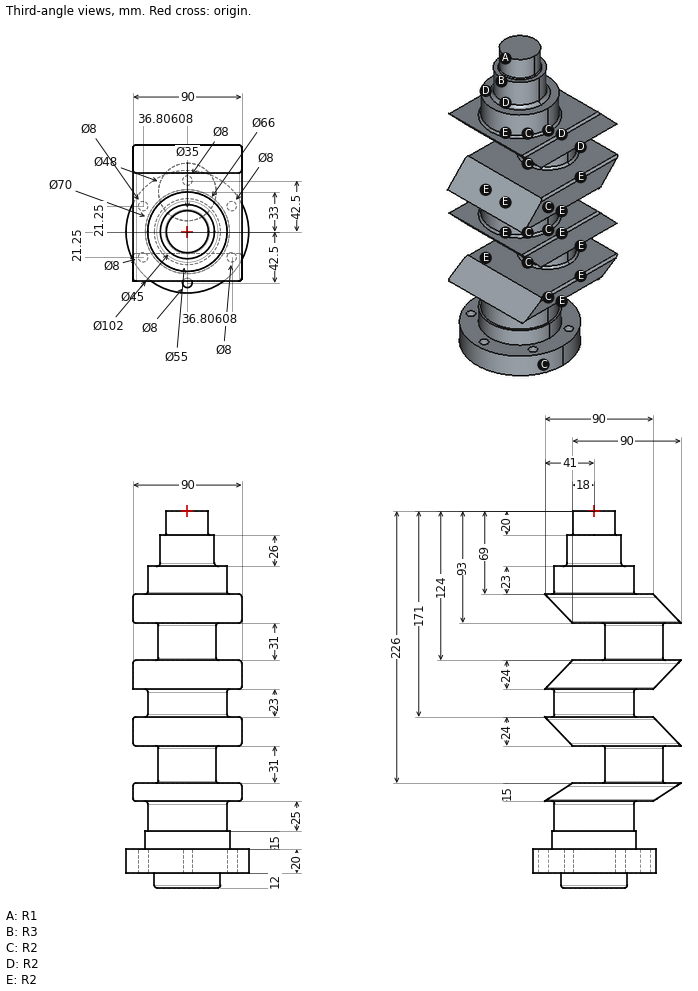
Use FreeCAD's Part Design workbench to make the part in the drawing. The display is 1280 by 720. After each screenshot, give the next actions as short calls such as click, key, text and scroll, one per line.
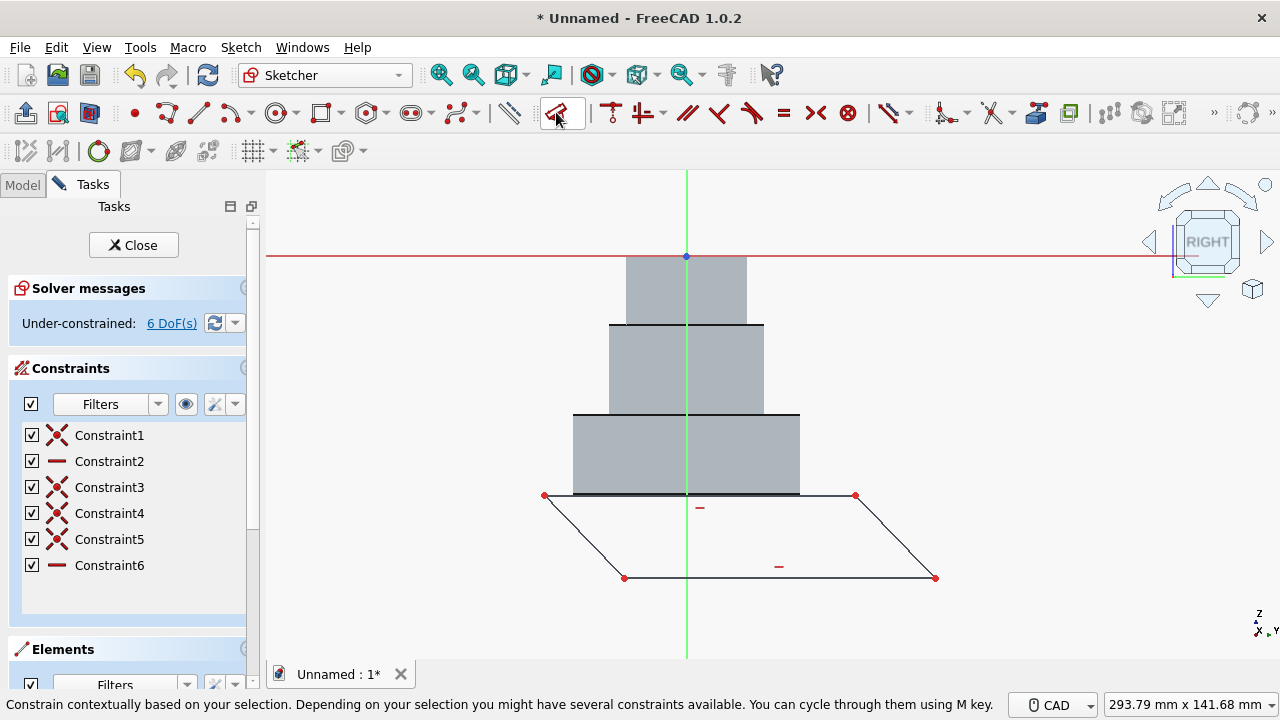
click(718, 578)
click(780, 612)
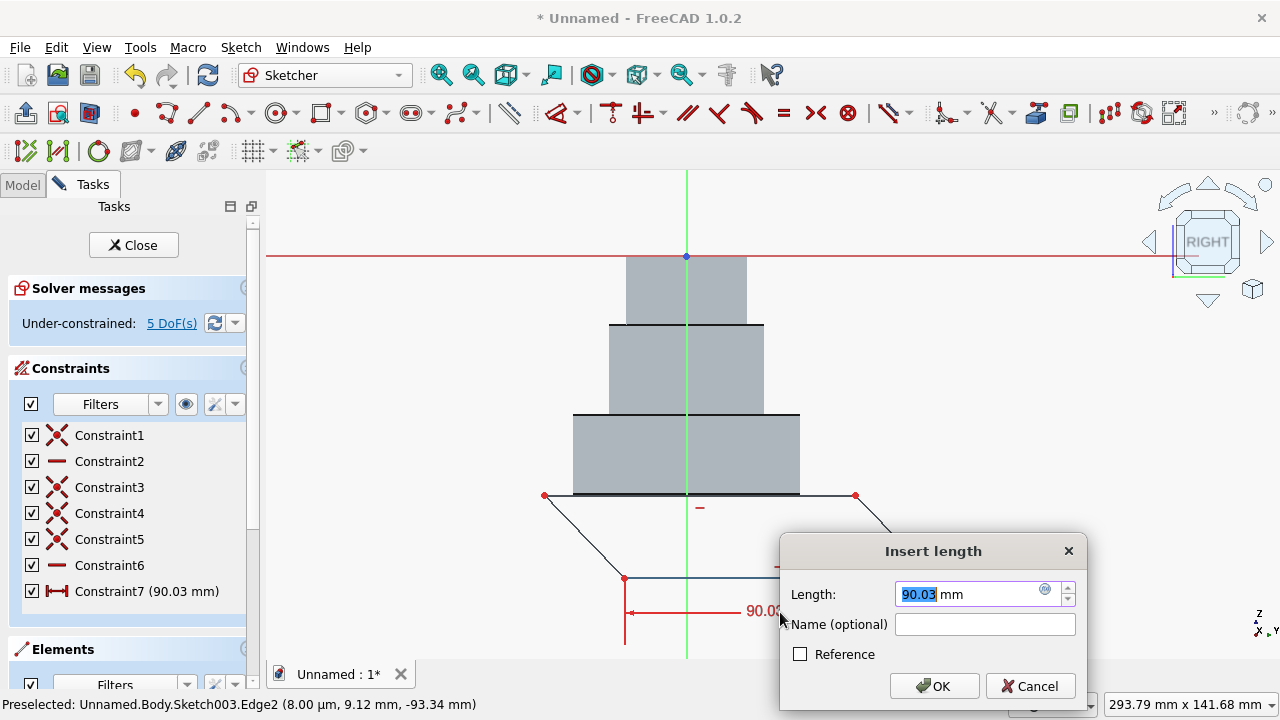
text(90)
key(Return)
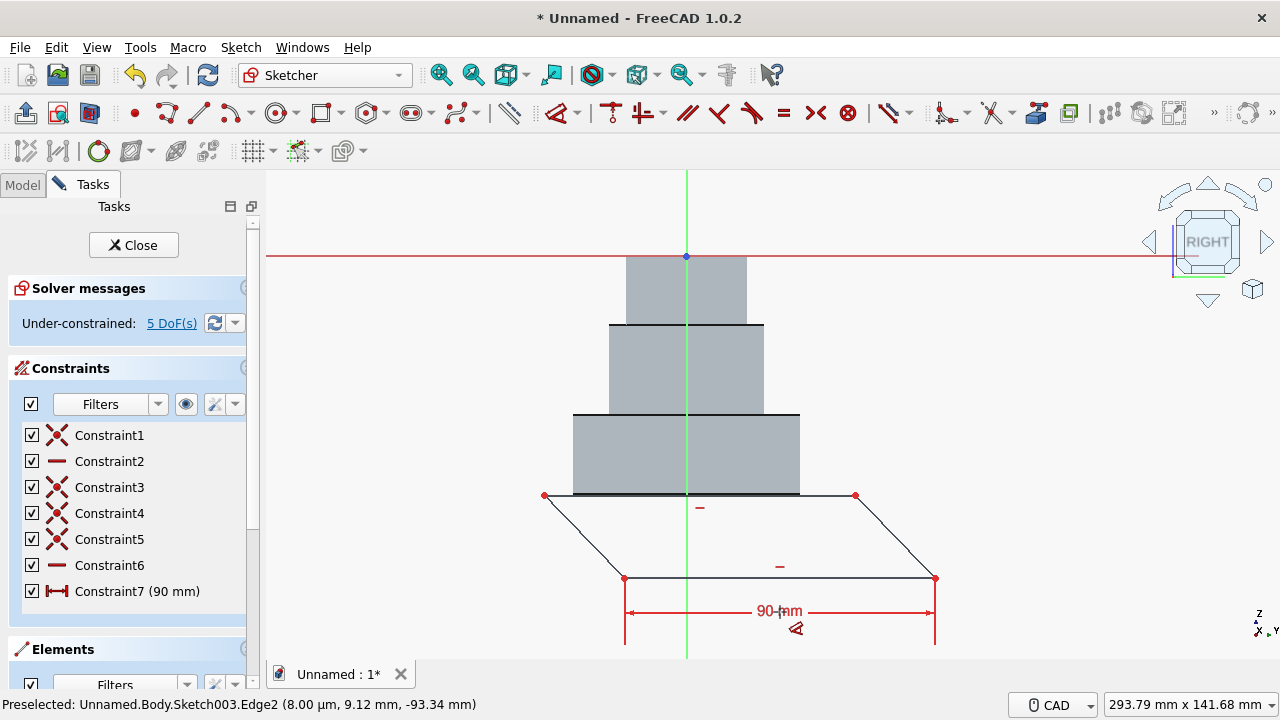
click(762, 496)
click(700, 530)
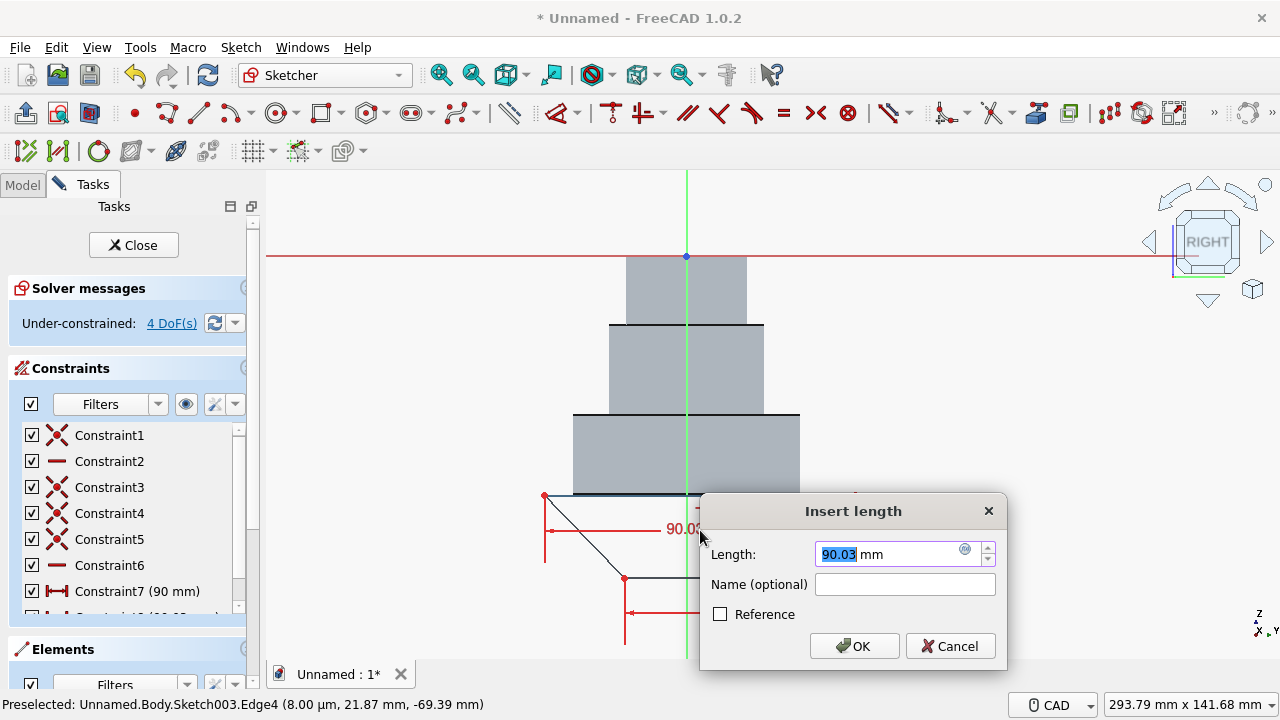
text(90)
key(Return)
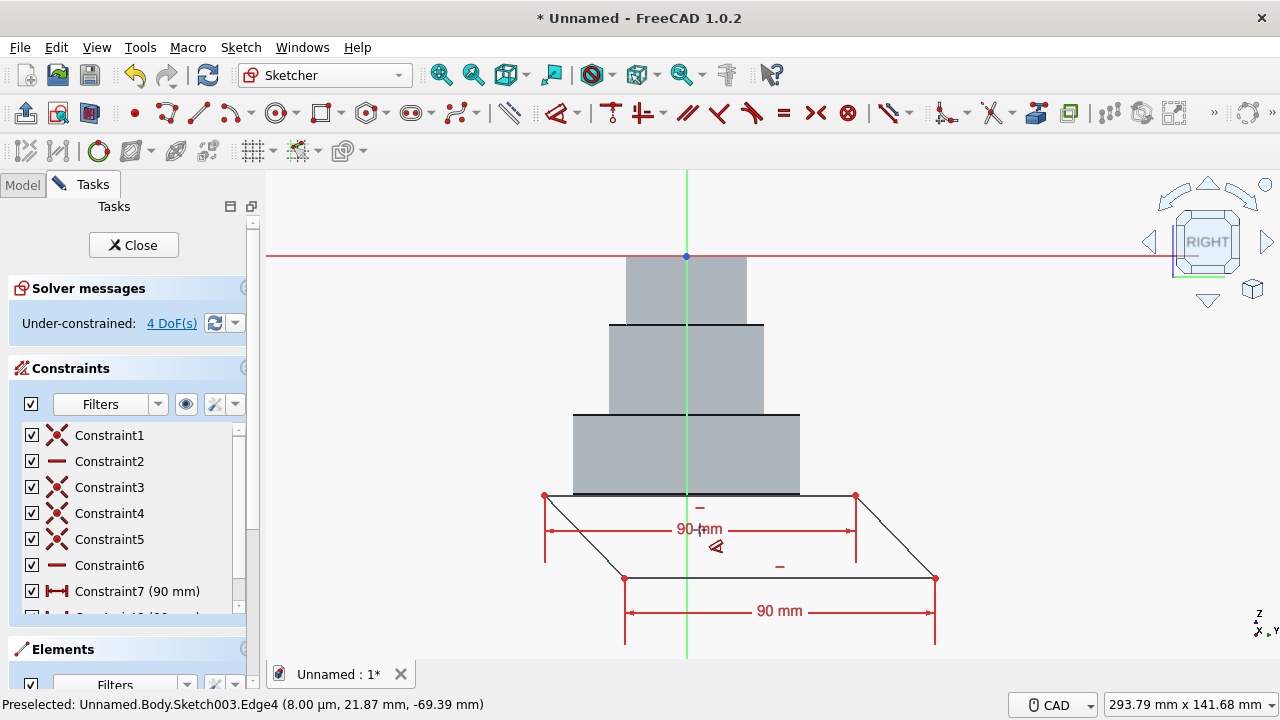
click(545, 496)
click(616, 222)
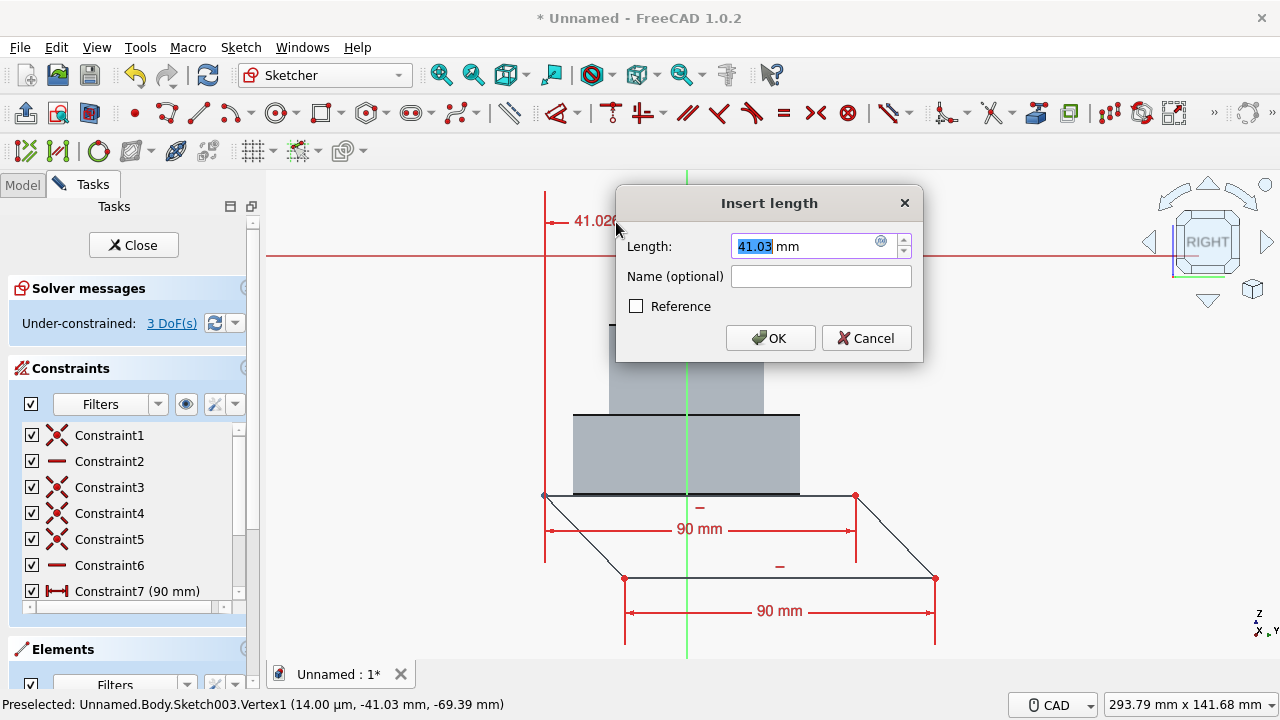
text(41)
key(Return)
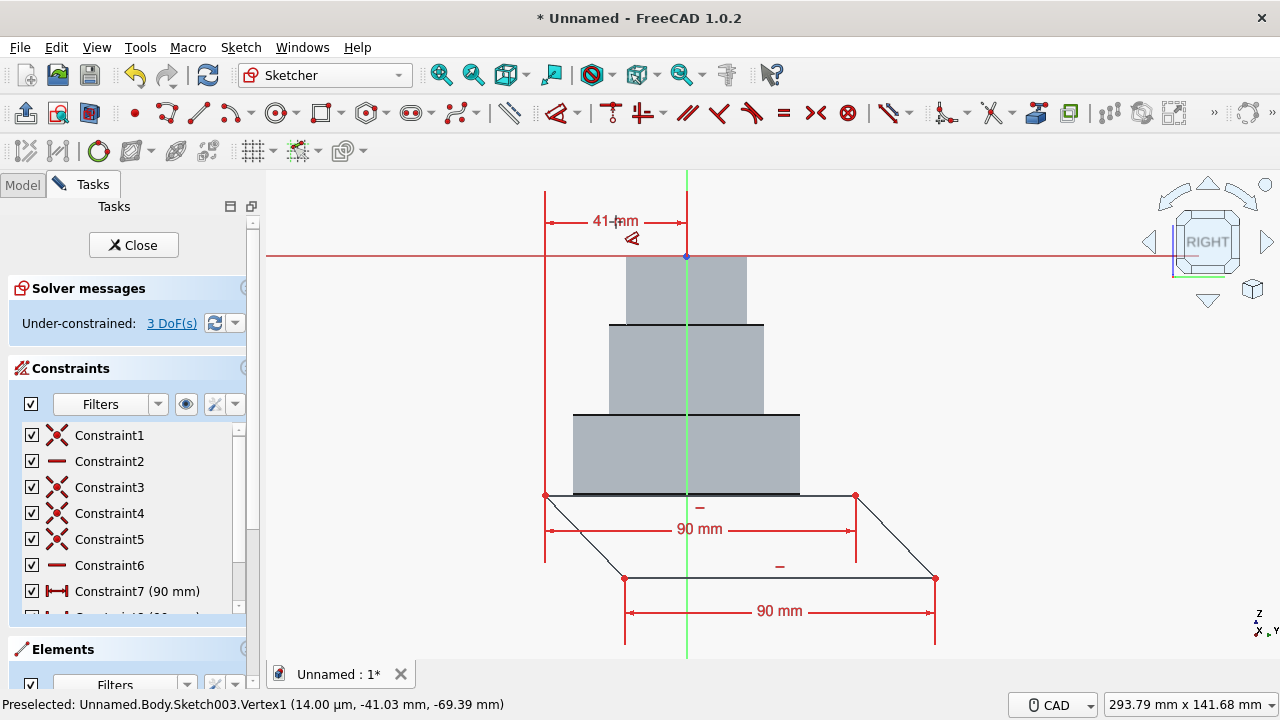
click(545, 496)
click(511, 376)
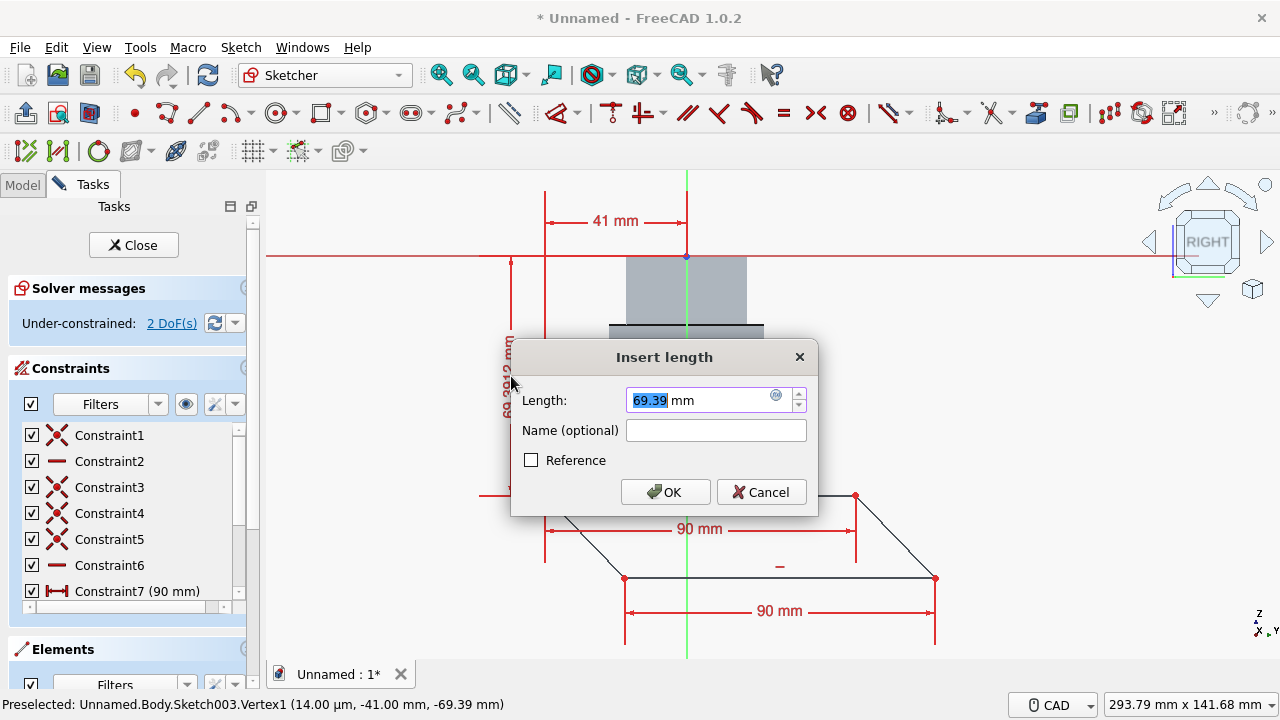
text(69)
key(Return)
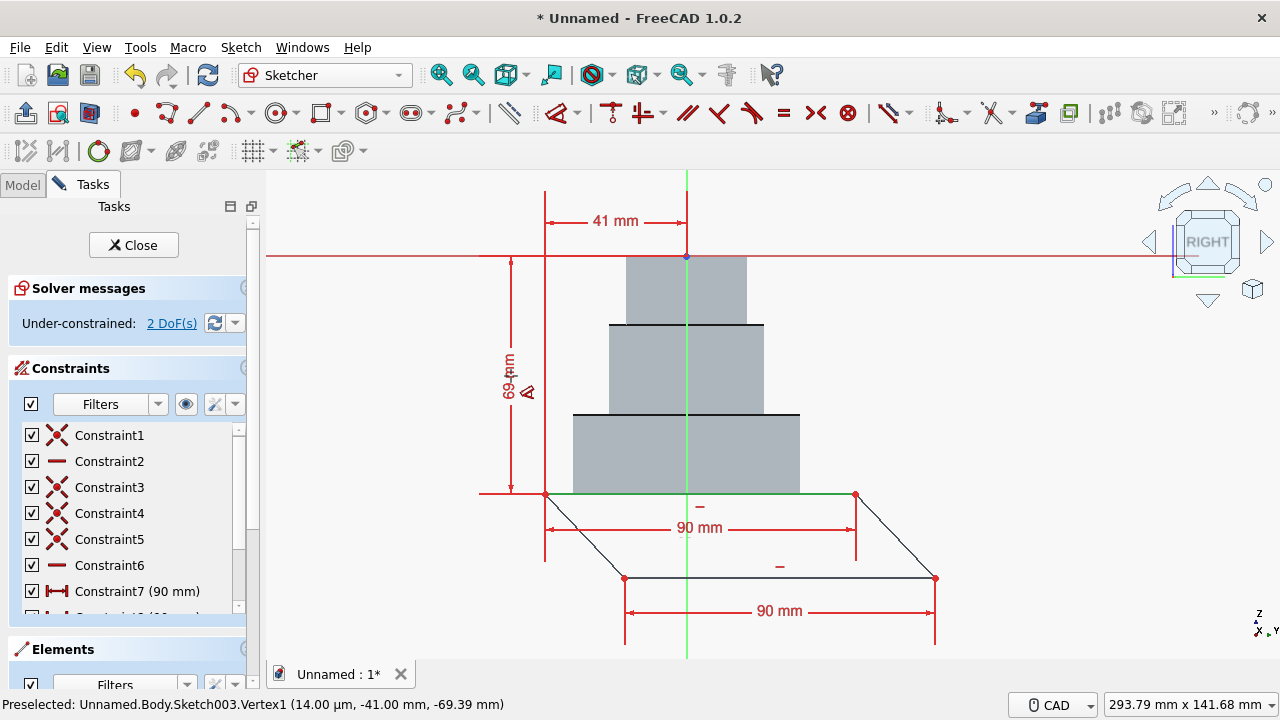
click(625, 578)
click(656, 612)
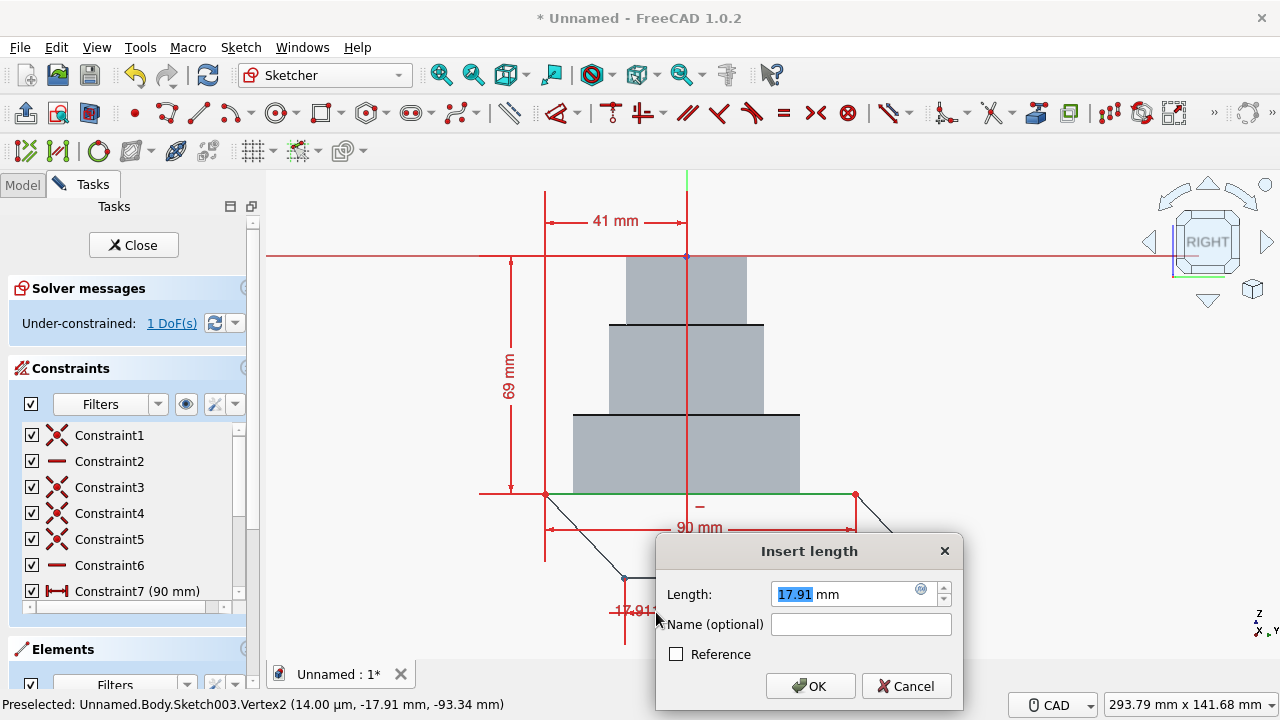
text(18)
key(Return)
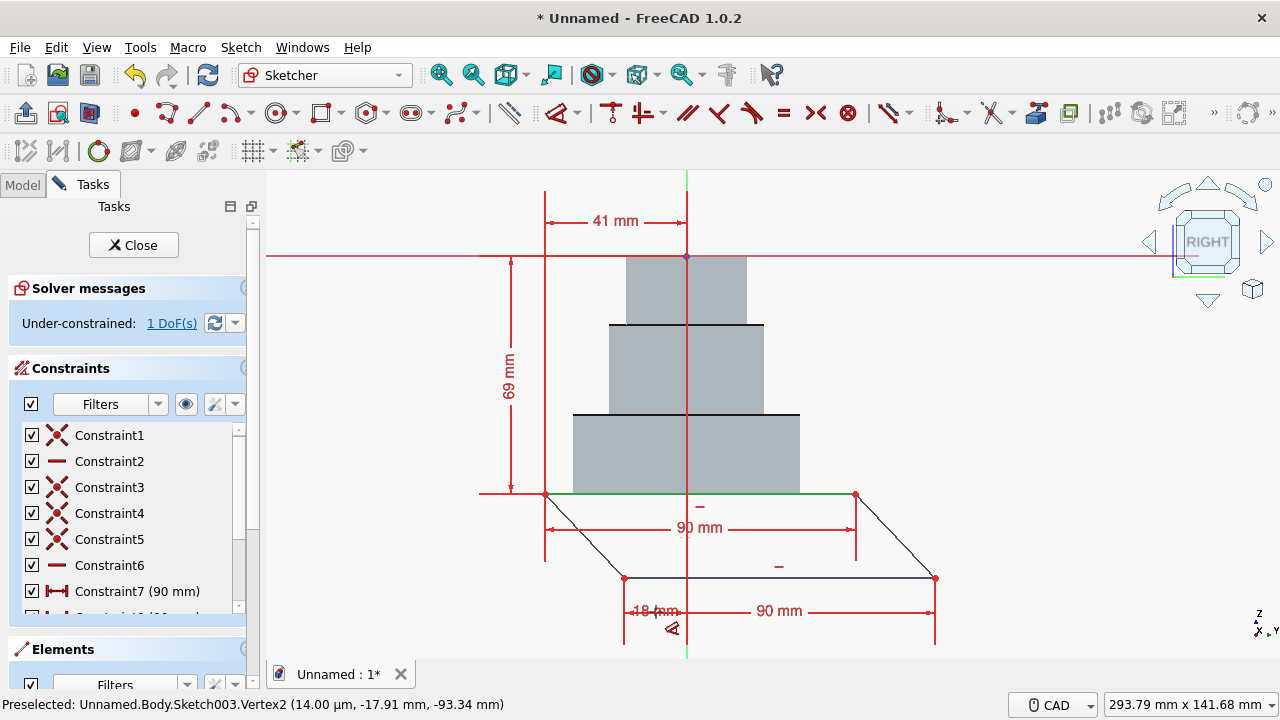
click(624, 578)
click(590, 417)